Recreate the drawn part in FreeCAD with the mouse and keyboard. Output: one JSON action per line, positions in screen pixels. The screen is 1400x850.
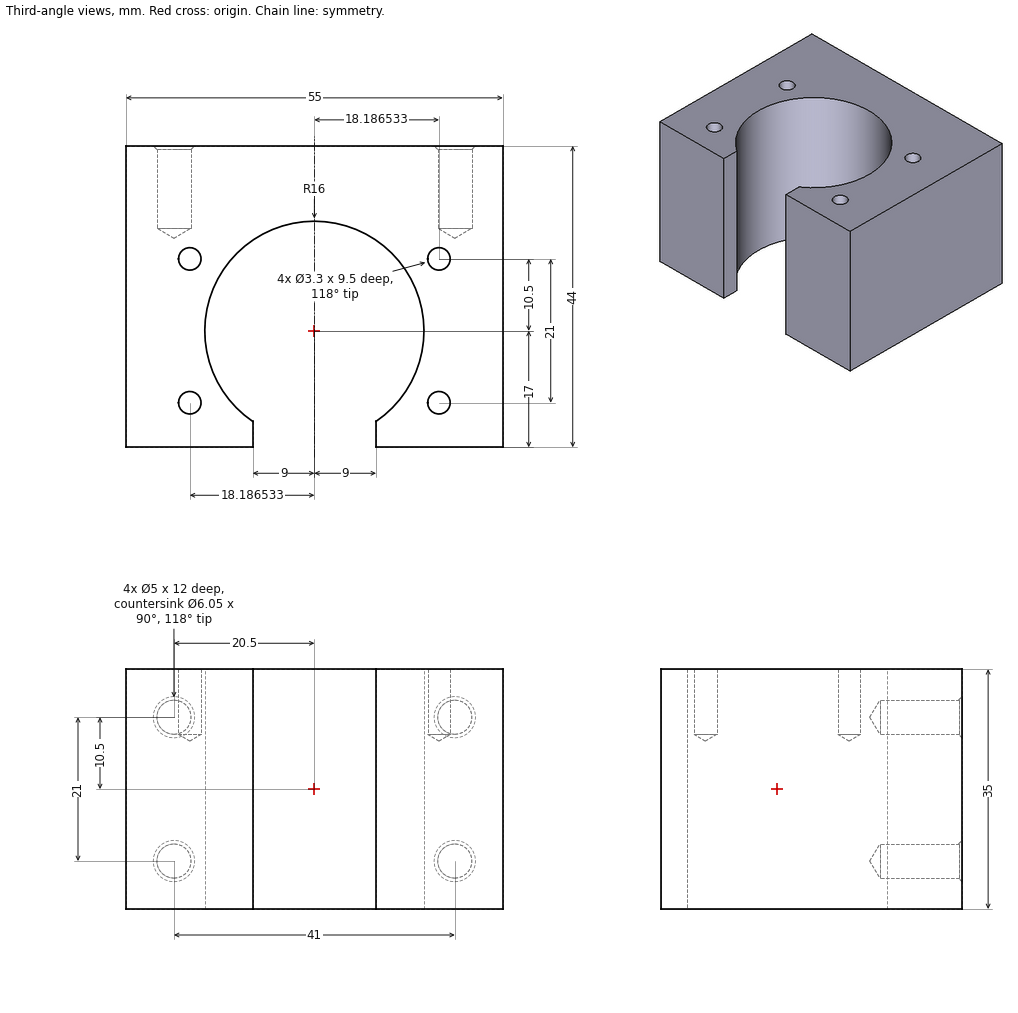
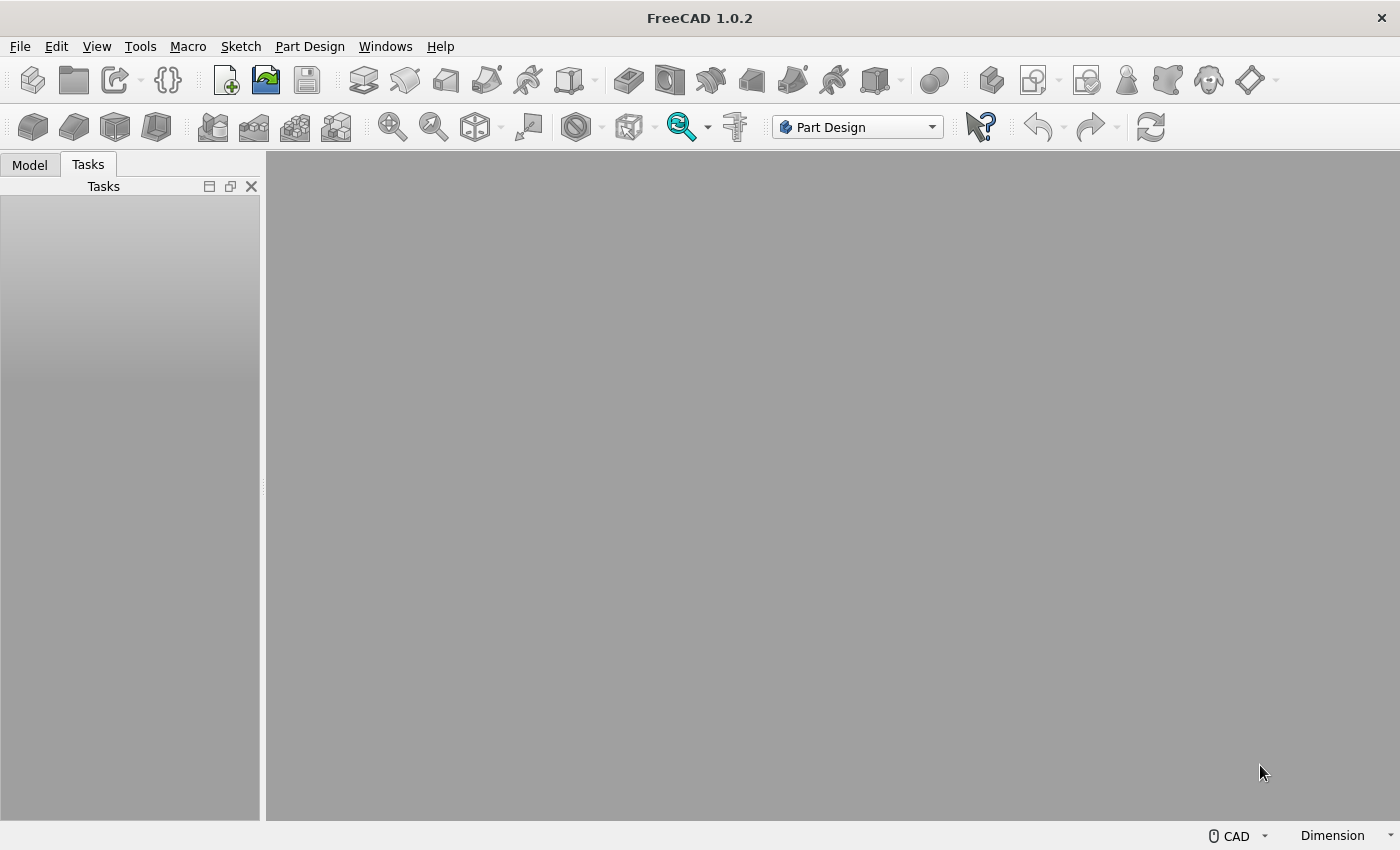
{"action": "left_click", "coordinate": [225, 80]}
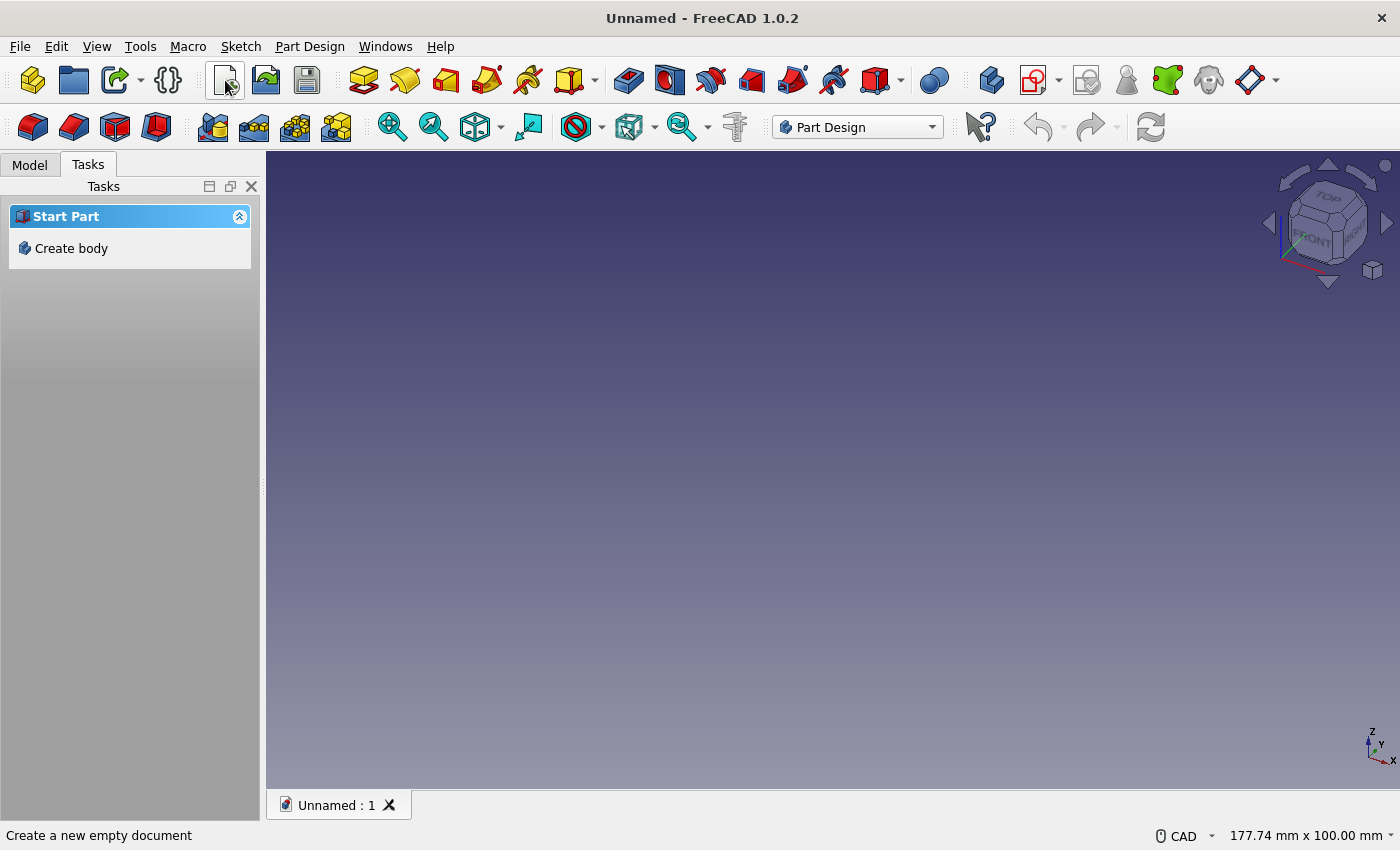
{"action": "left_click", "coordinate": [1032, 80]}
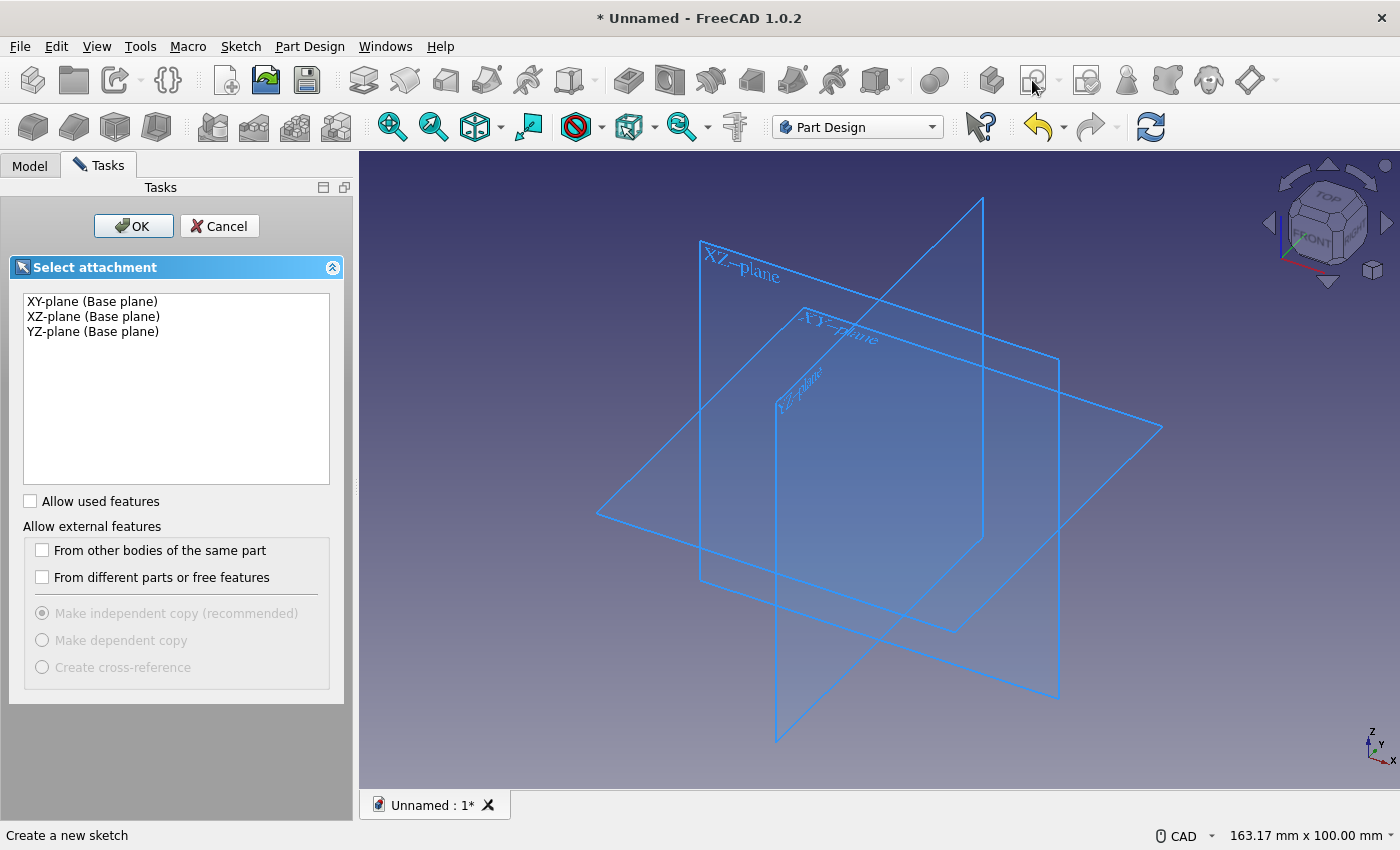
{"action": "left_click", "coordinate": [84, 302]}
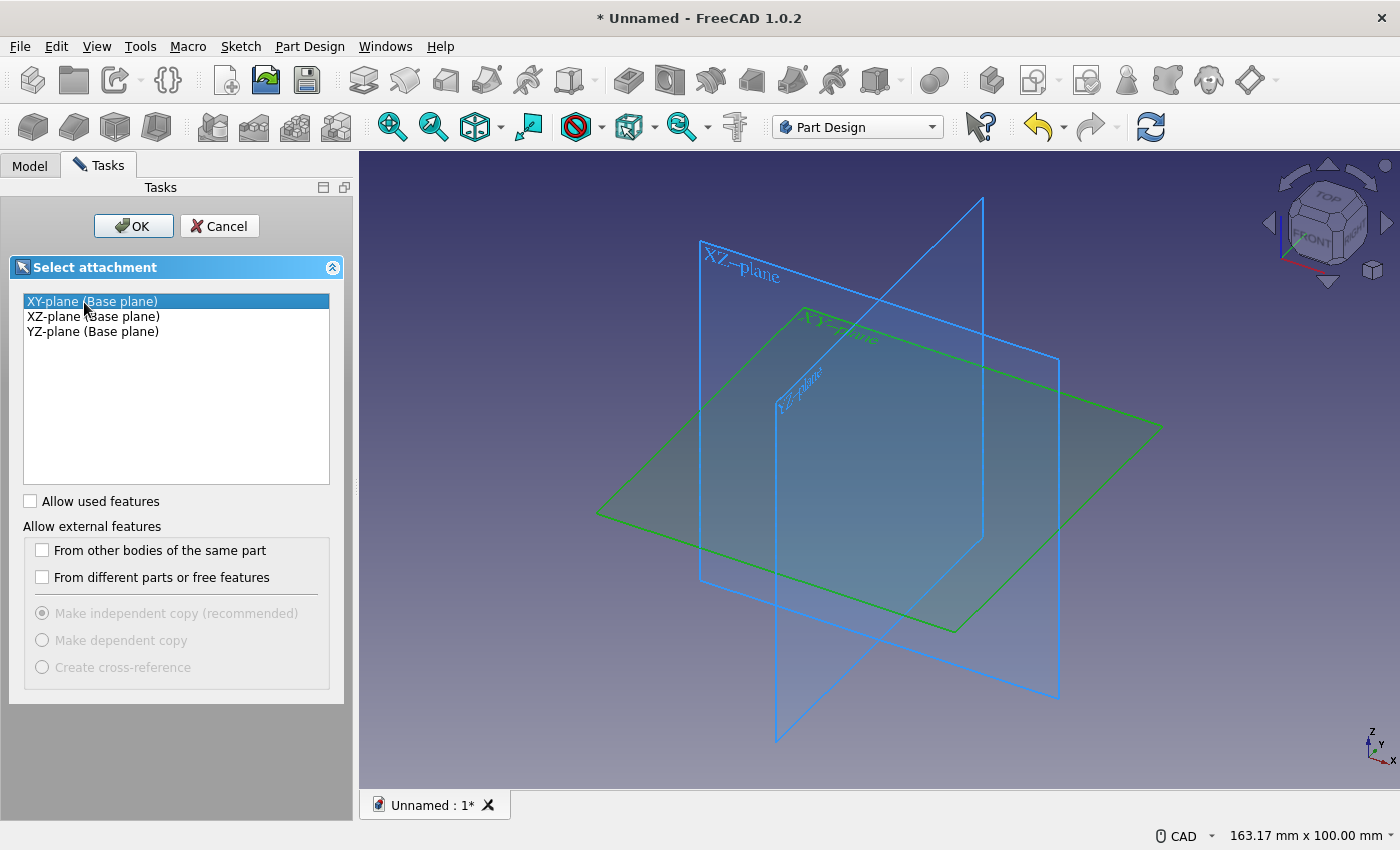
{"action": "left_click", "coordinate": [134, 226]}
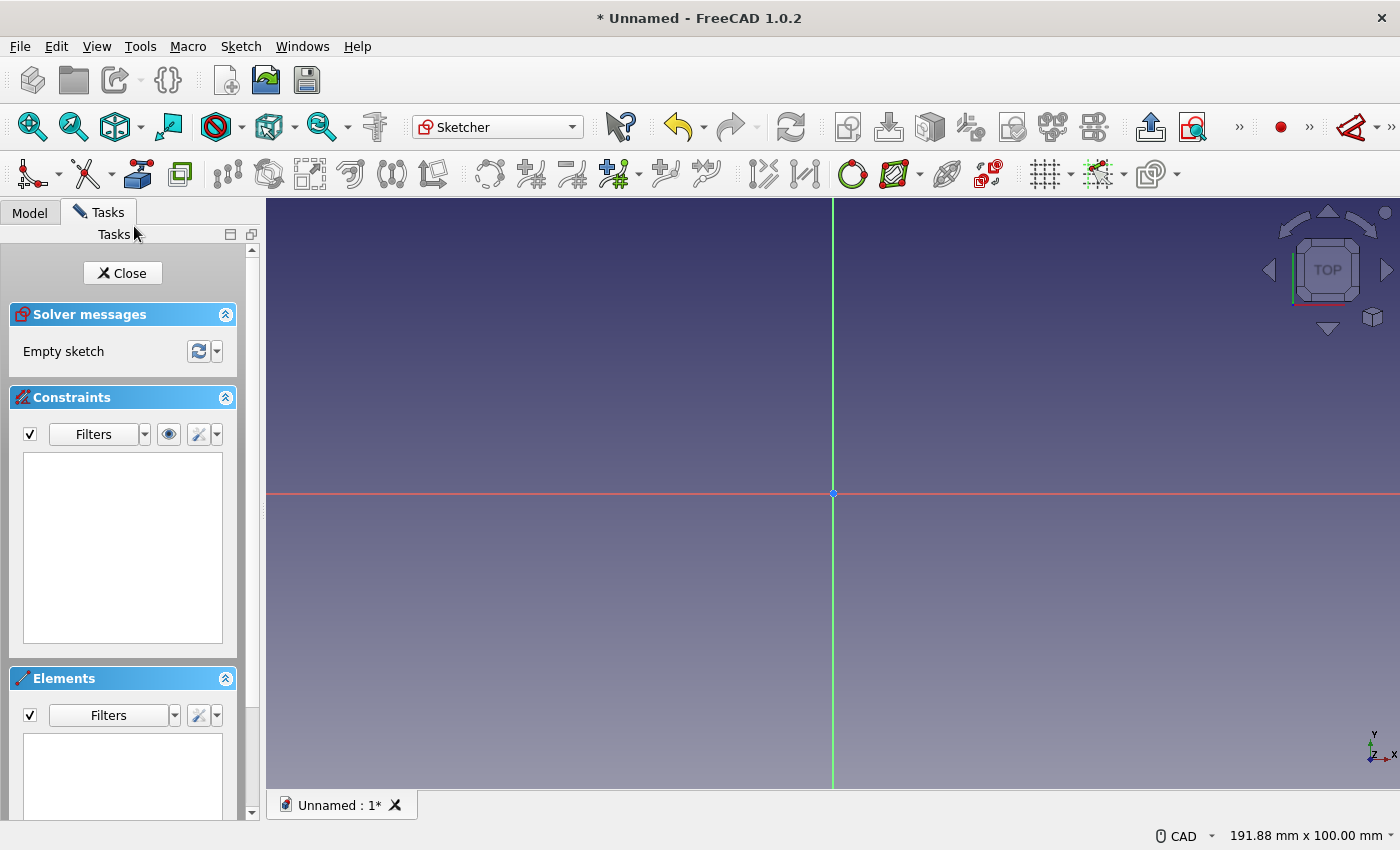
{"action": "scroll", "coordinate": [972, 404], "scroll_direction": "up", "scroll_amount": 2}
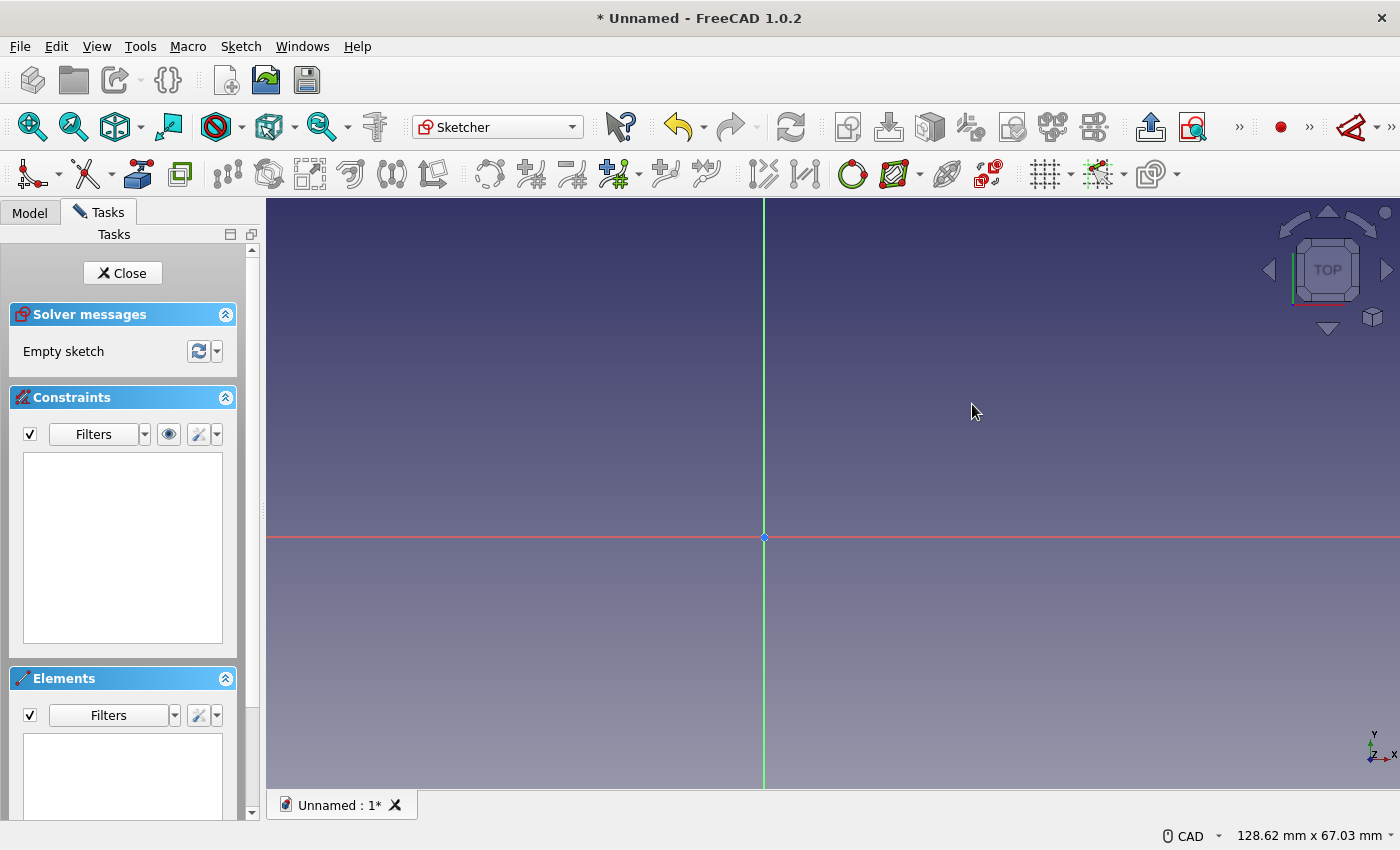
{"action": "key", "text": "g m"}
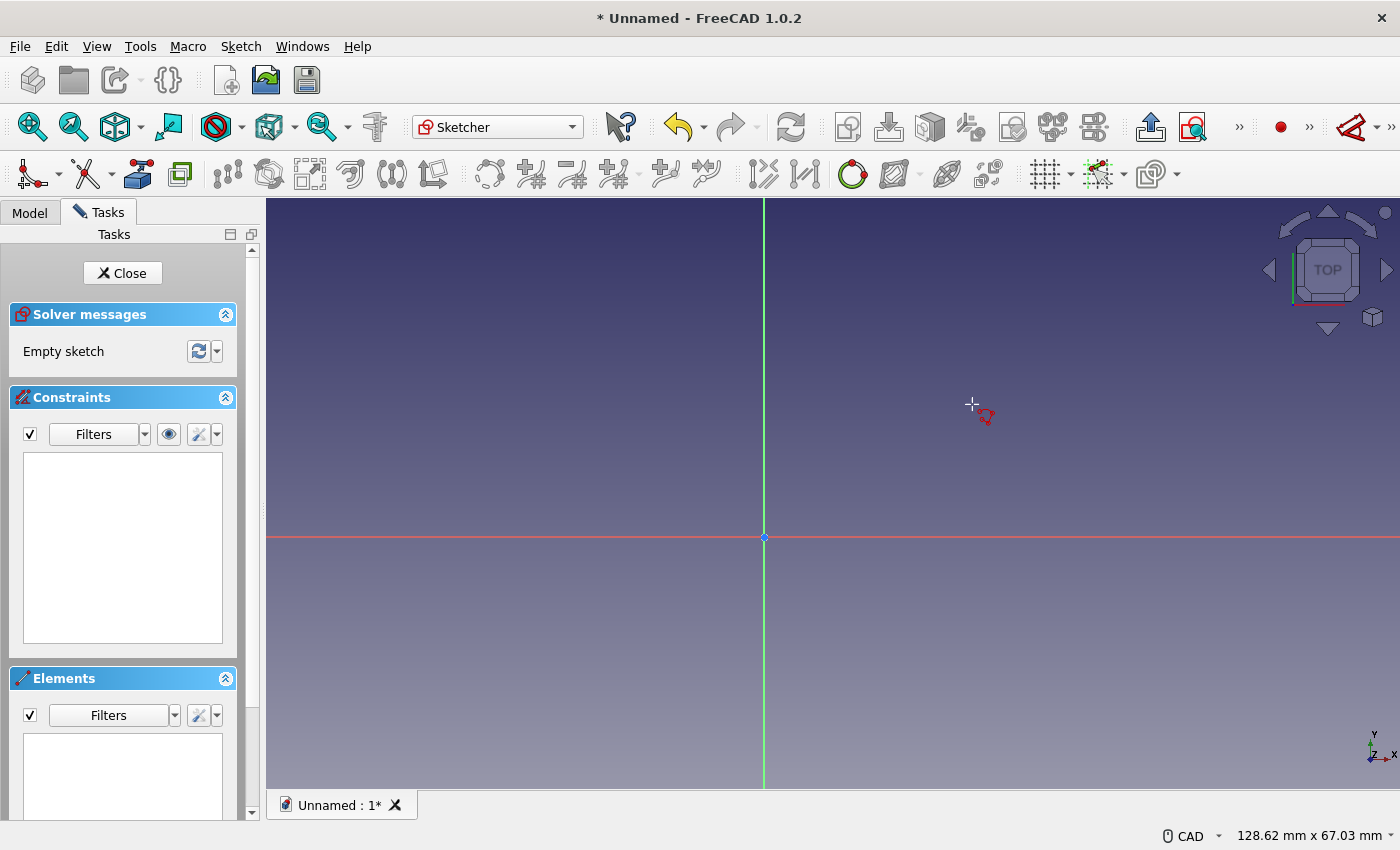
{"action": "left_click", "coordinate": [844, 654]}
{"action": "left_click", "coordinate": [844, 687]}
{"action": "left_click", "coordinate": [1007, 687]}
{"action": "left_click", "coordinate": [1007, 299]}
{"action": "left_click", "coordinate": [522, 299]}
{"action": "left_click", "coordinate": [522, 687]}
{"action": "left_click", "coordinate": [685, 687]}
{"action": "left_click", "coordinate": [685, 654]}
{"action": "right_click", "coordinate": [685, 654]}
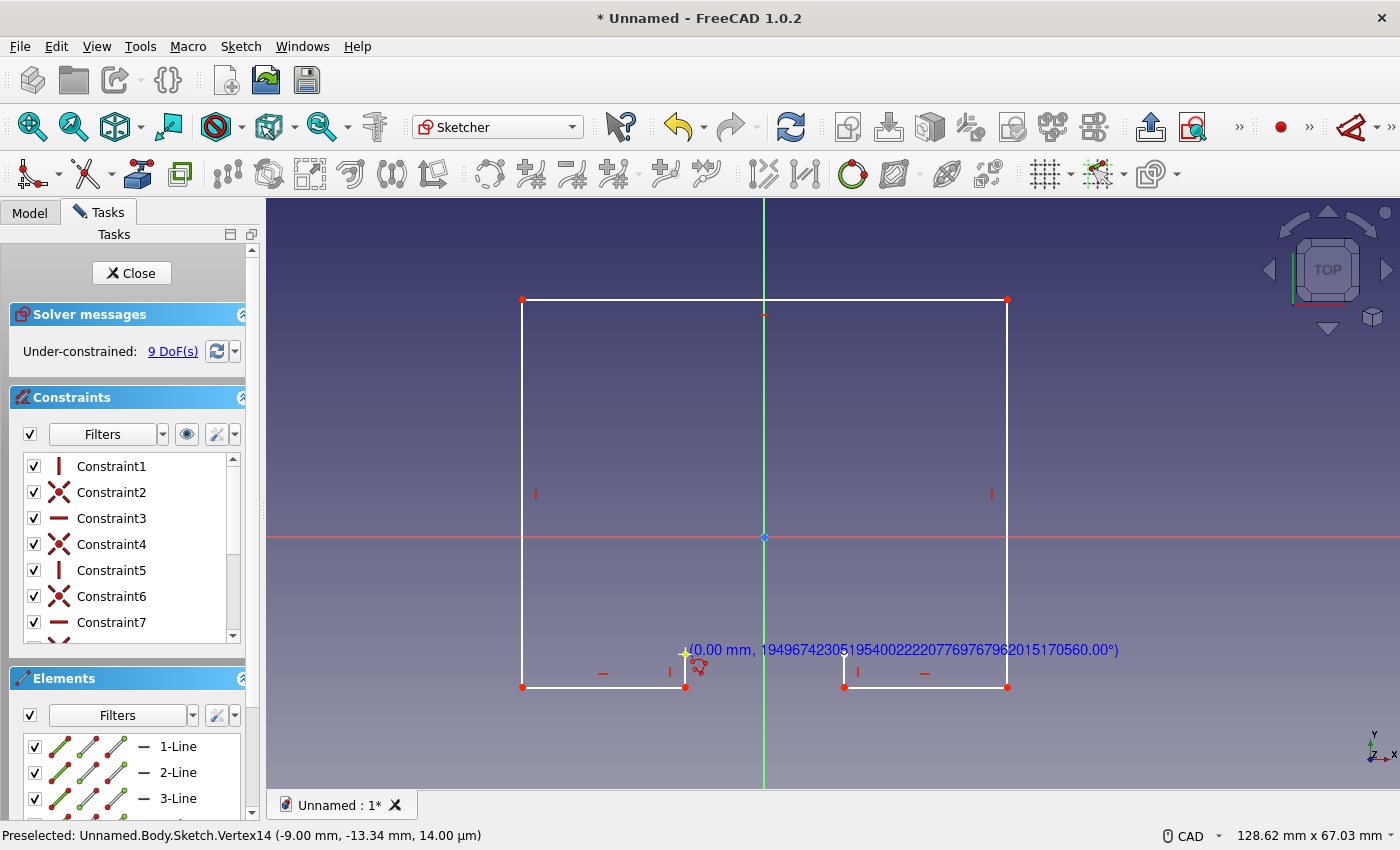
{"action": "key", "text": "g 3 a"}